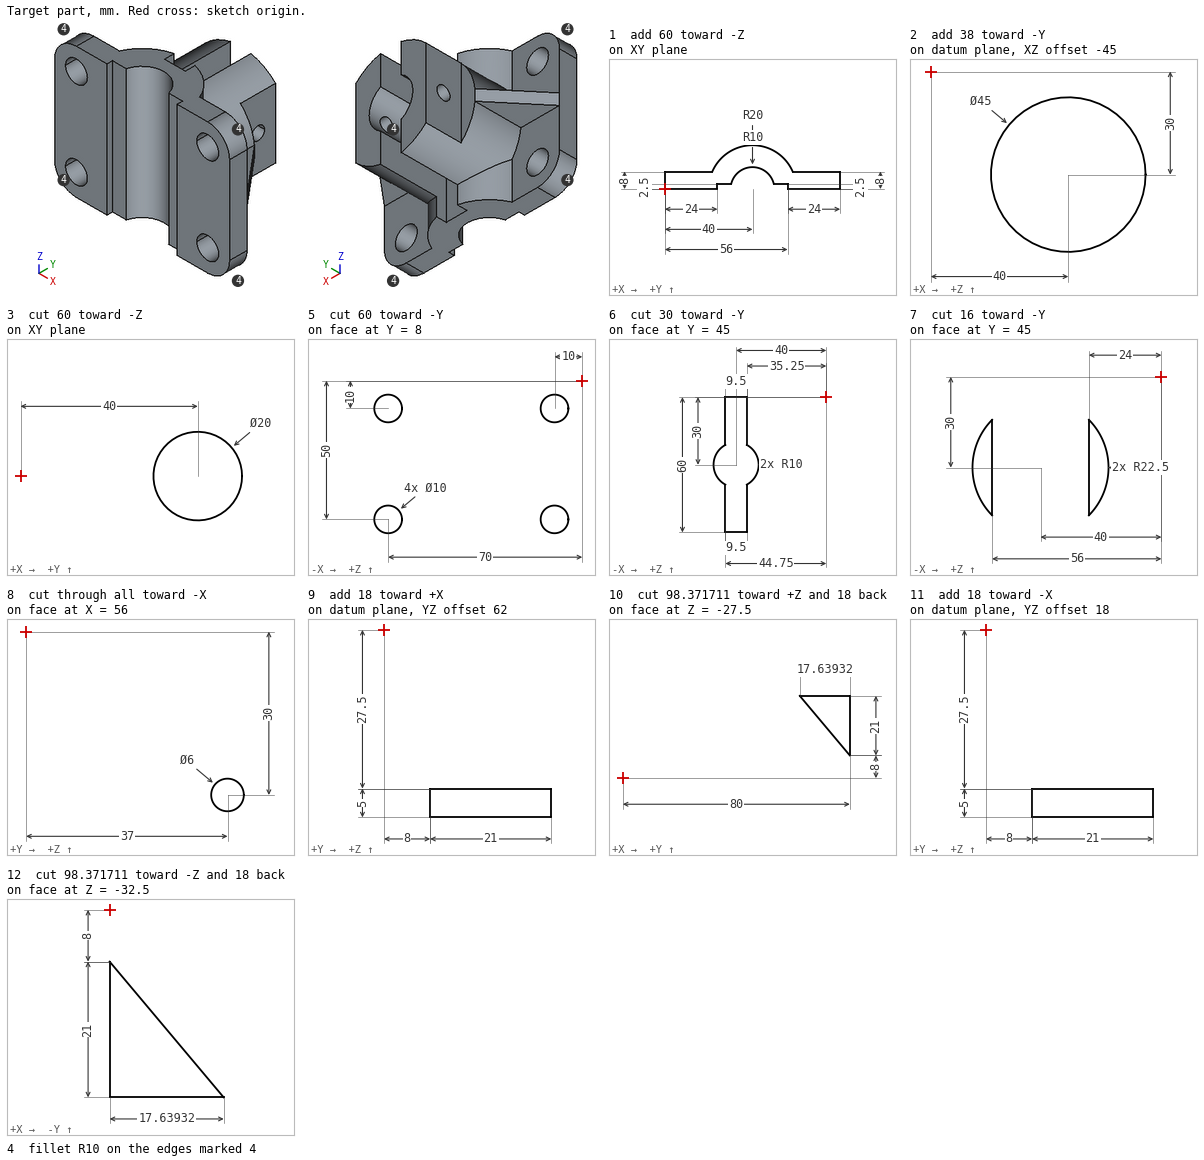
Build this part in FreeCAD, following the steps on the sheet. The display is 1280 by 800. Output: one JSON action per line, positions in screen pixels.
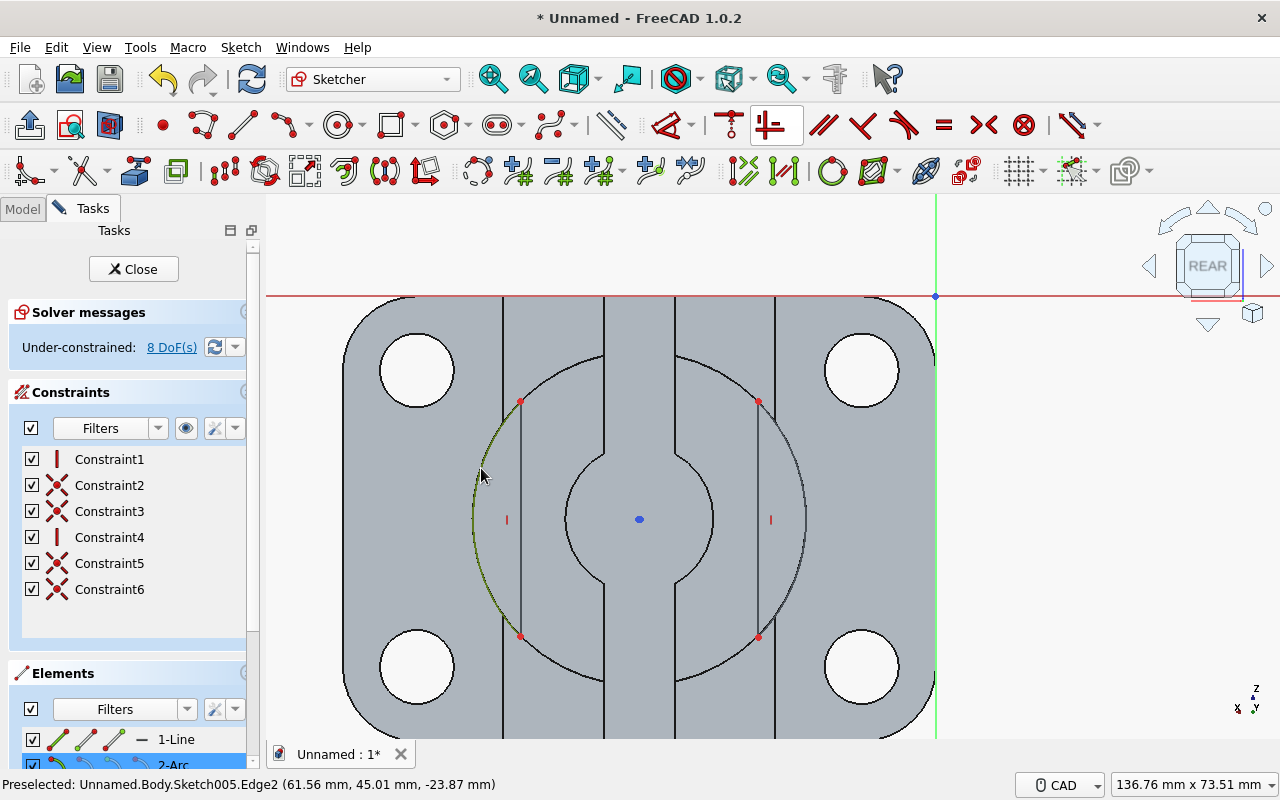
{"action": "left_click", "coordinate": [798, 571]}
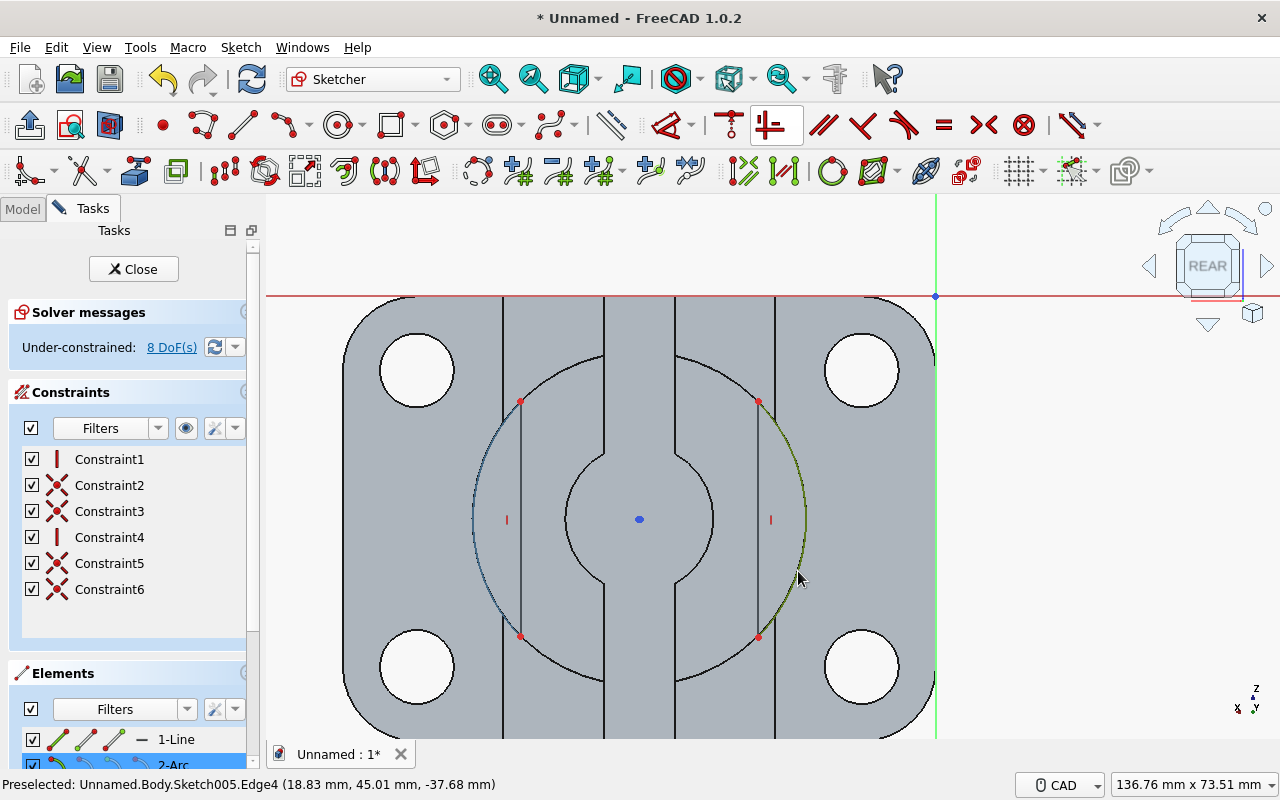
{"action": "left_click", "coordinate": [730, 126]}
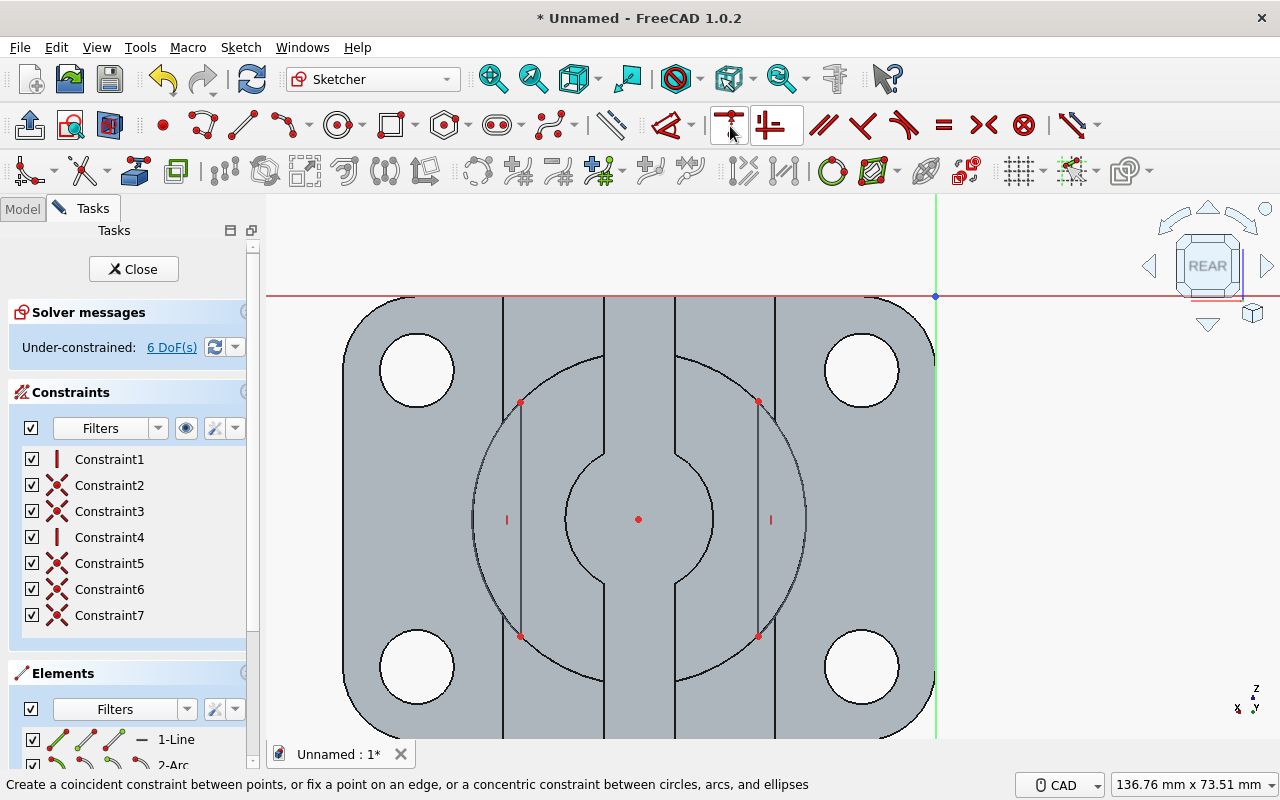
{"action": "left_click", "coordinate": [480, 468]}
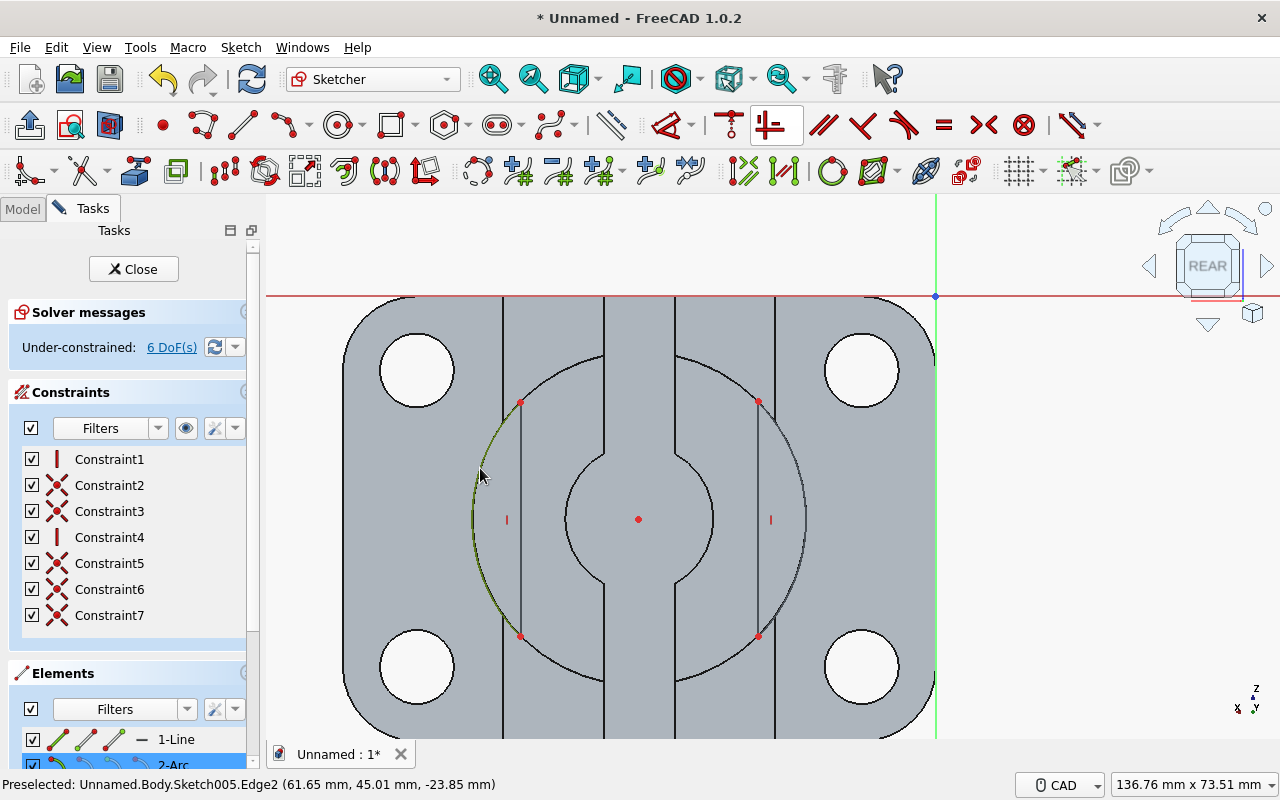
{"action": "left_click", "coordinate": [798, 571]}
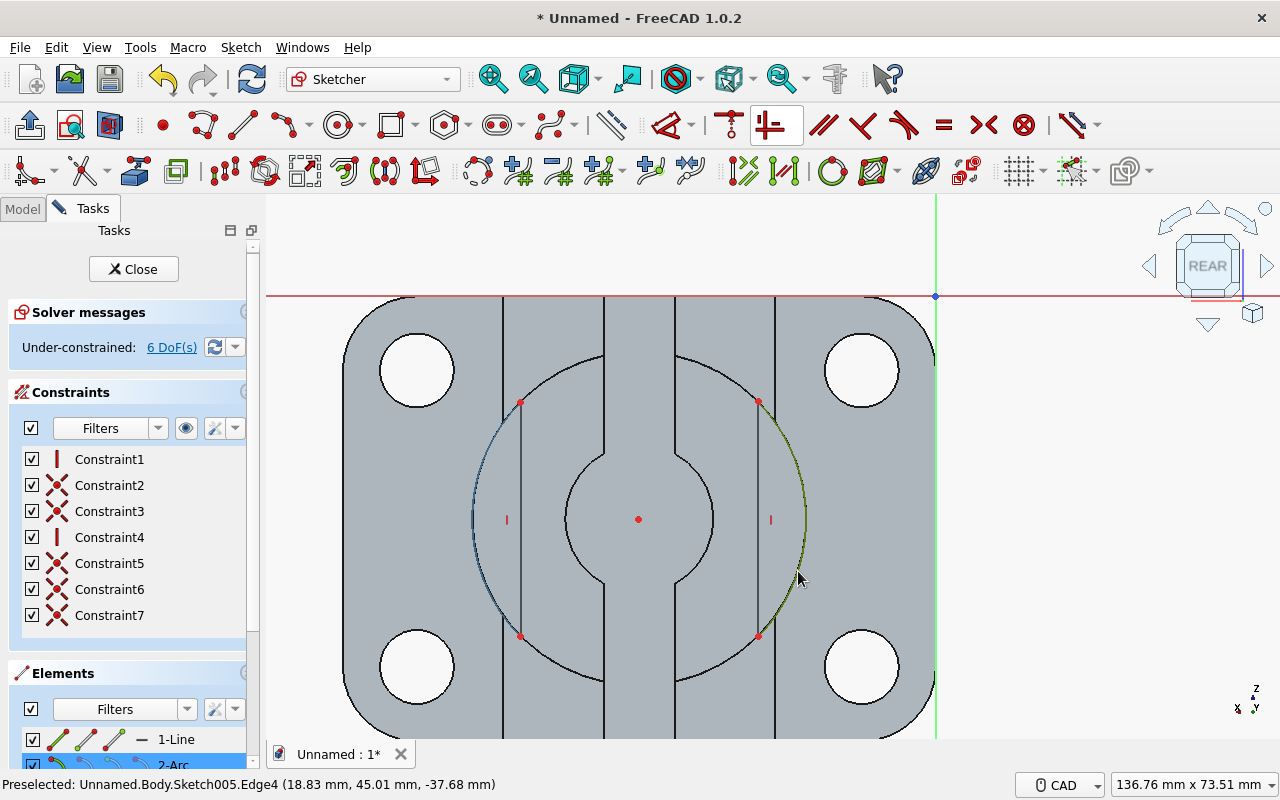
{"action": "left_click", "coordinate": [944, 126]}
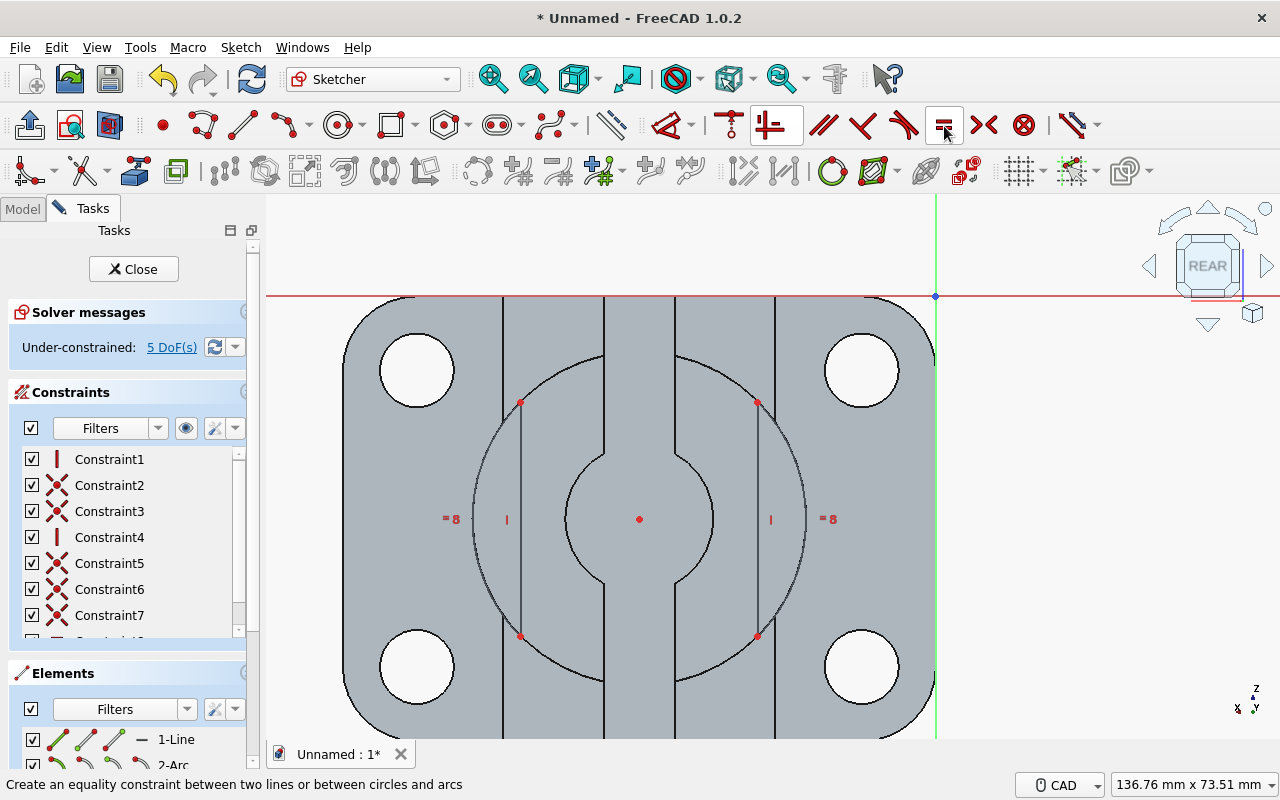
{"action": "left_click", "coordinate": [666, 126]}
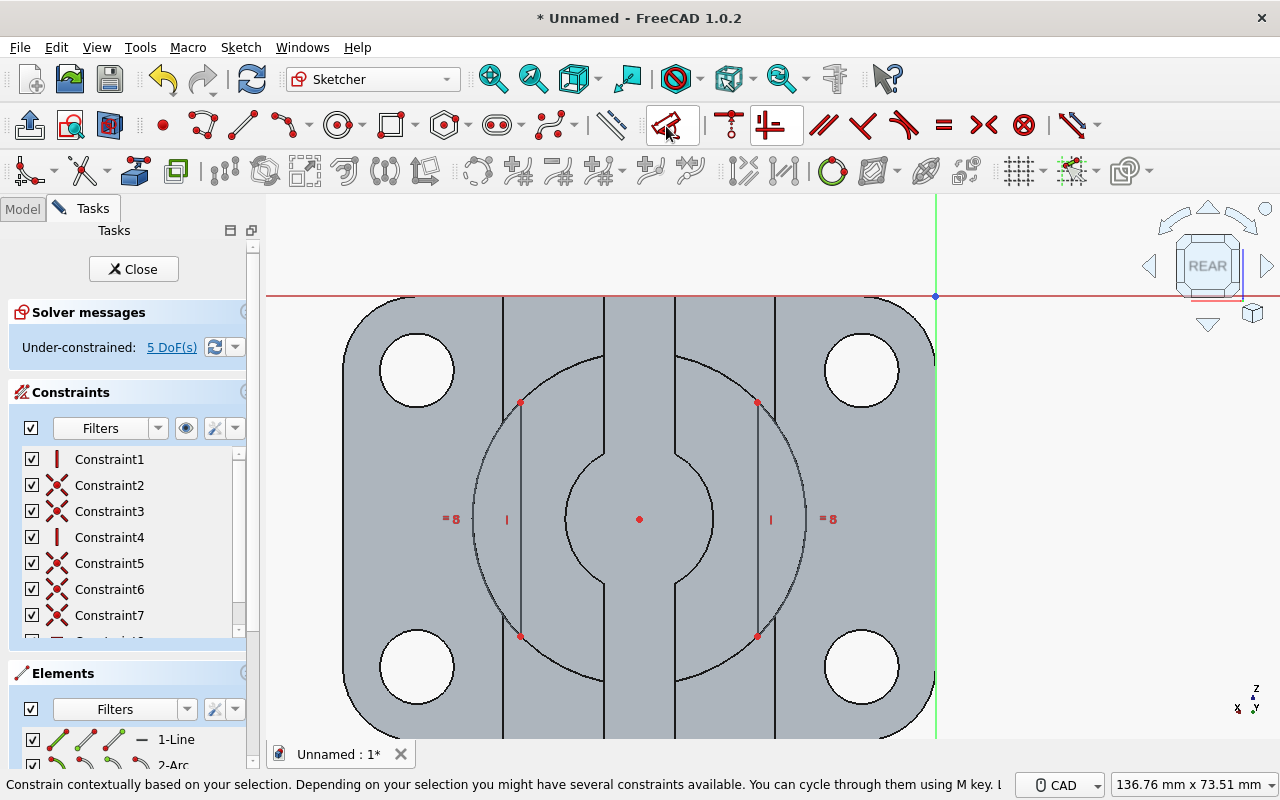
{"action": "left_click", "coordinate": [481, 468]}
{"action": "left_click", "coordinate": [451, 458]}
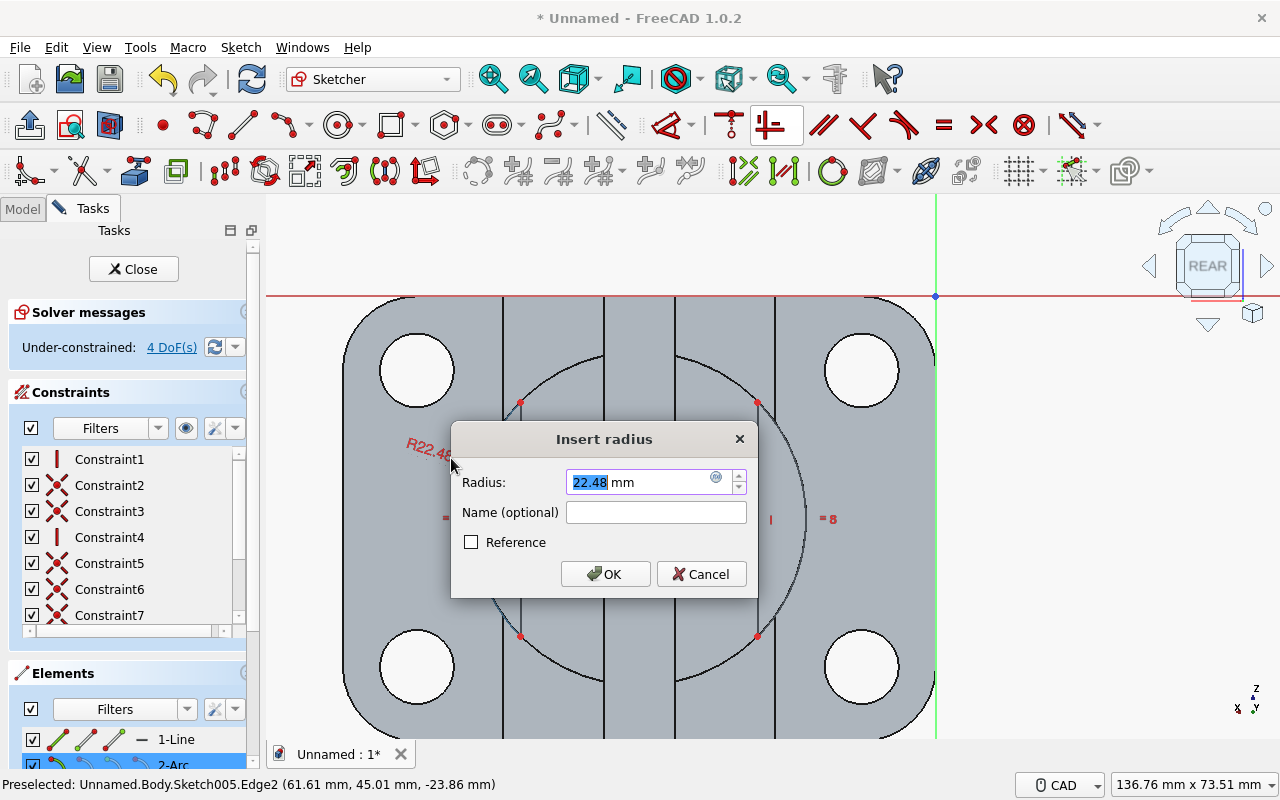
{"action": "type", "text": "22.5"}
{"action": "key", "text": "Return"}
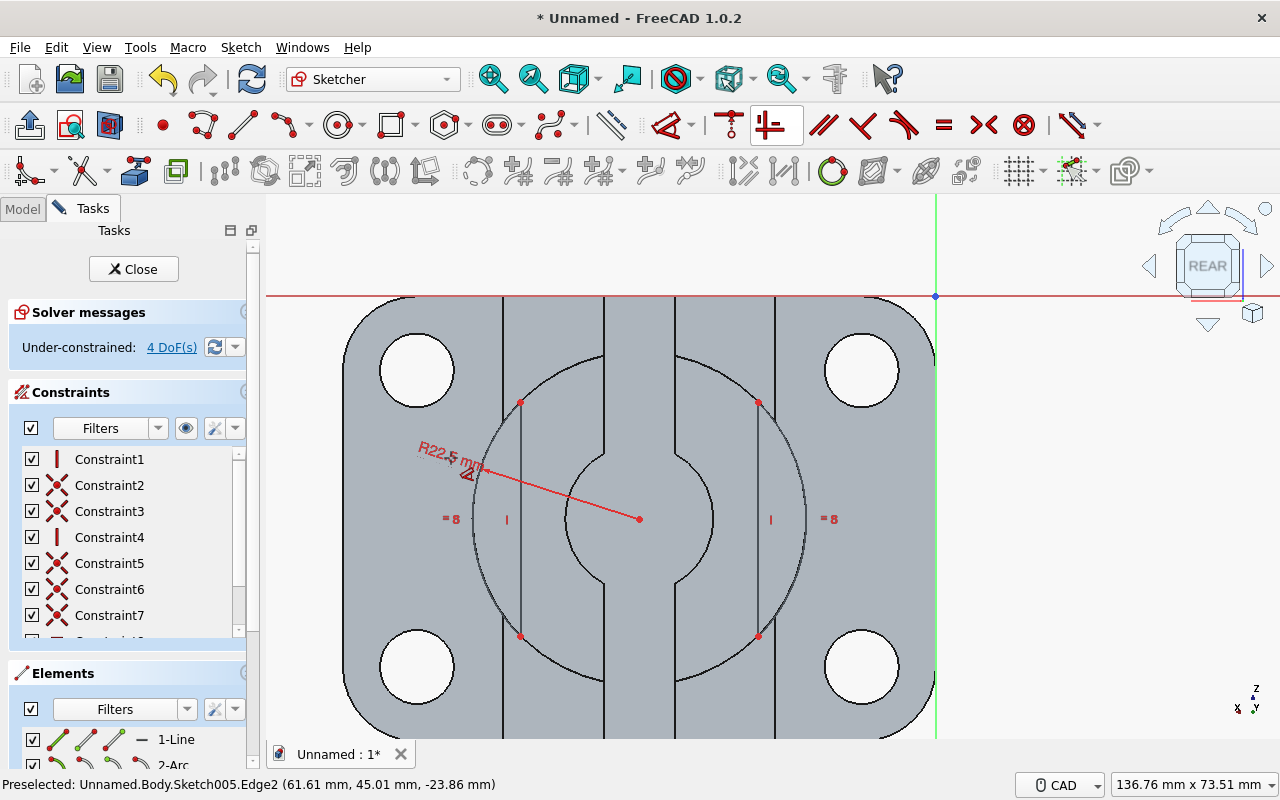
{"action": "left_click", "coordinate": [521, 637]}
{"action": "left_click", "coordinate": [728, 671]}